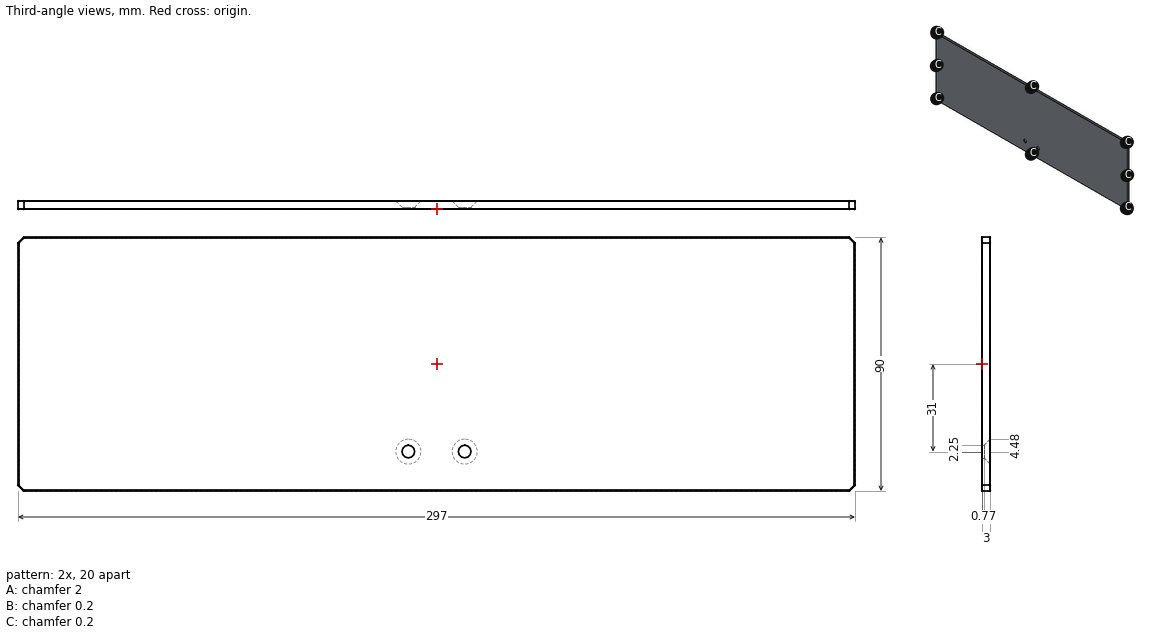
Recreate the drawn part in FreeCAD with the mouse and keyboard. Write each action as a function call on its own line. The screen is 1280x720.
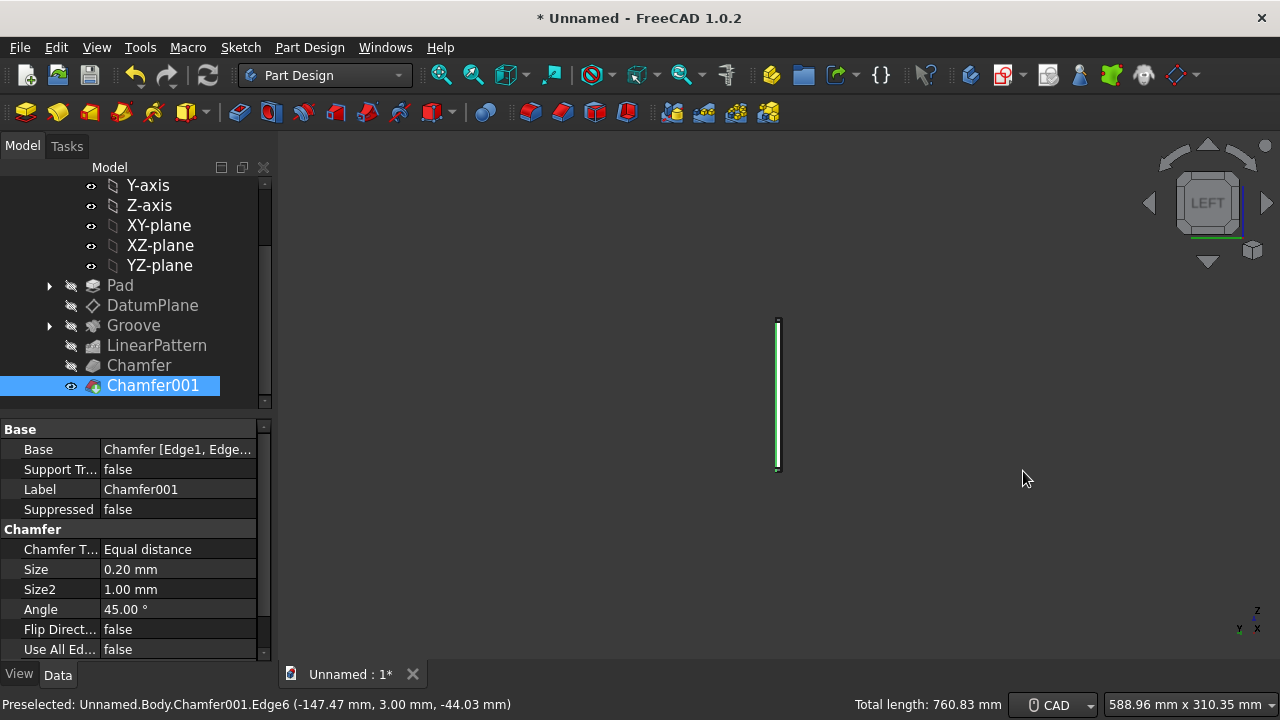
scroll(776, 319, up, 11)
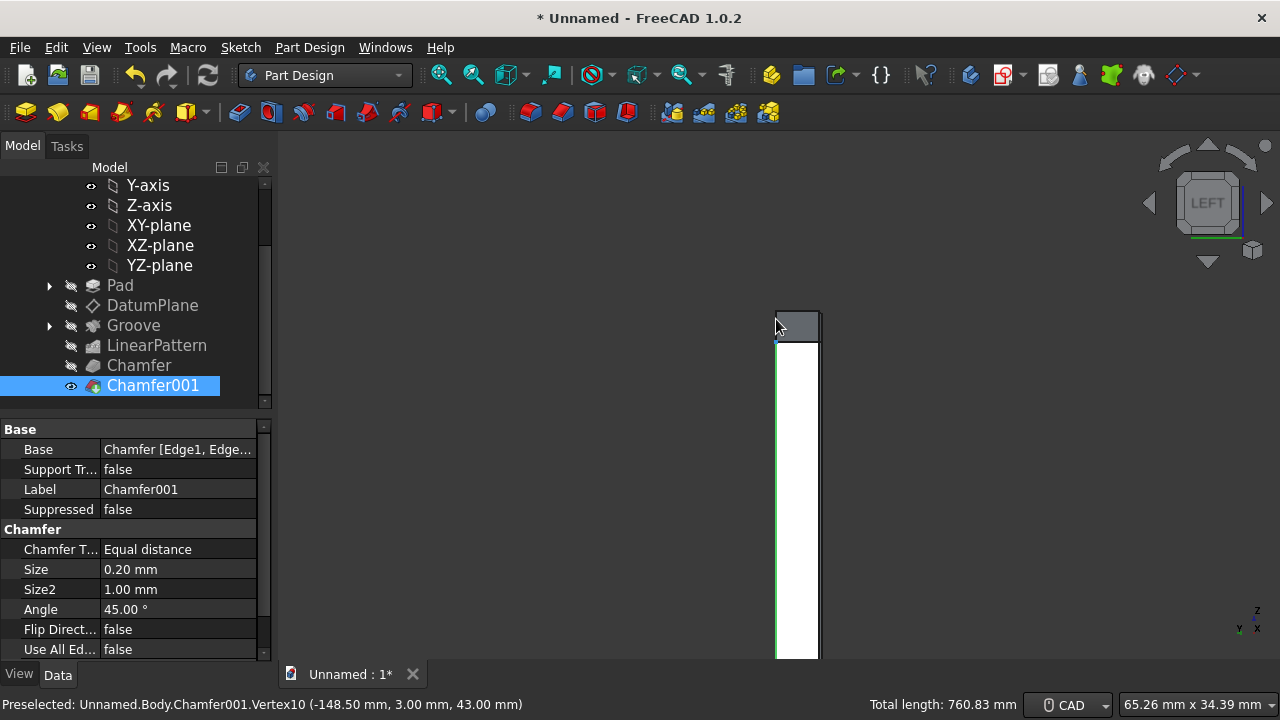
click(776, 325, ctrl)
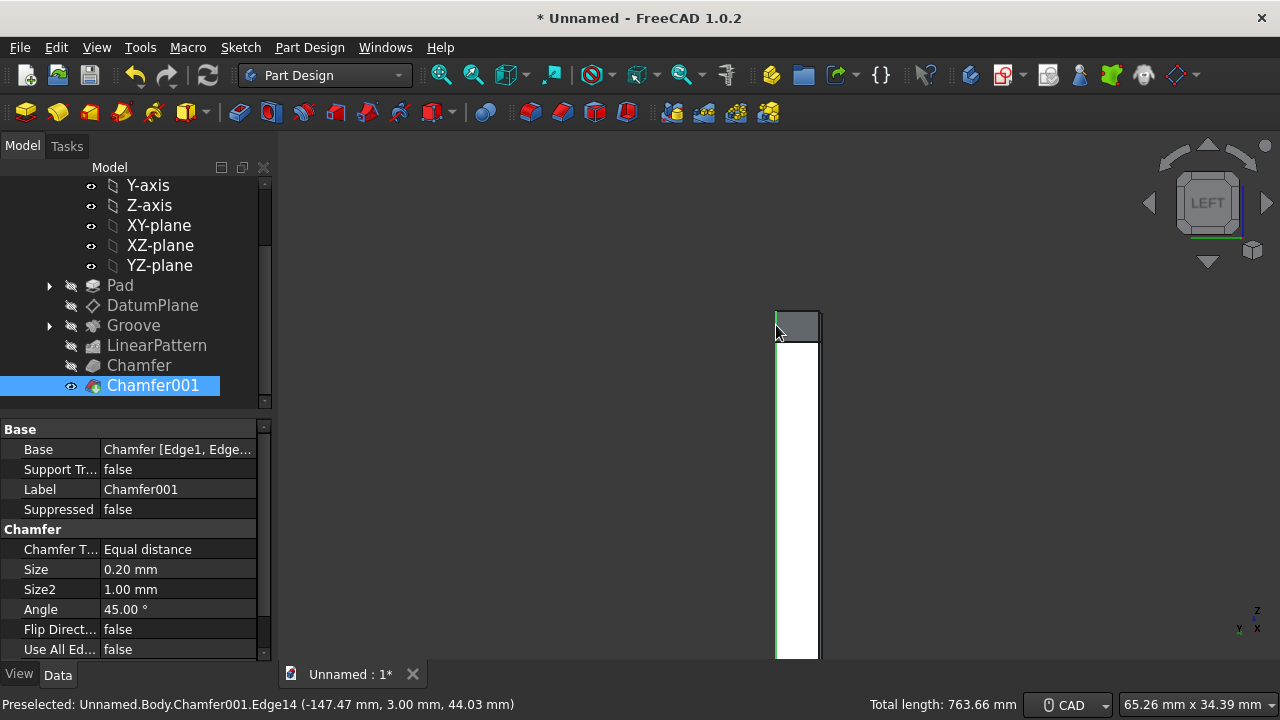
key(v)
key(f)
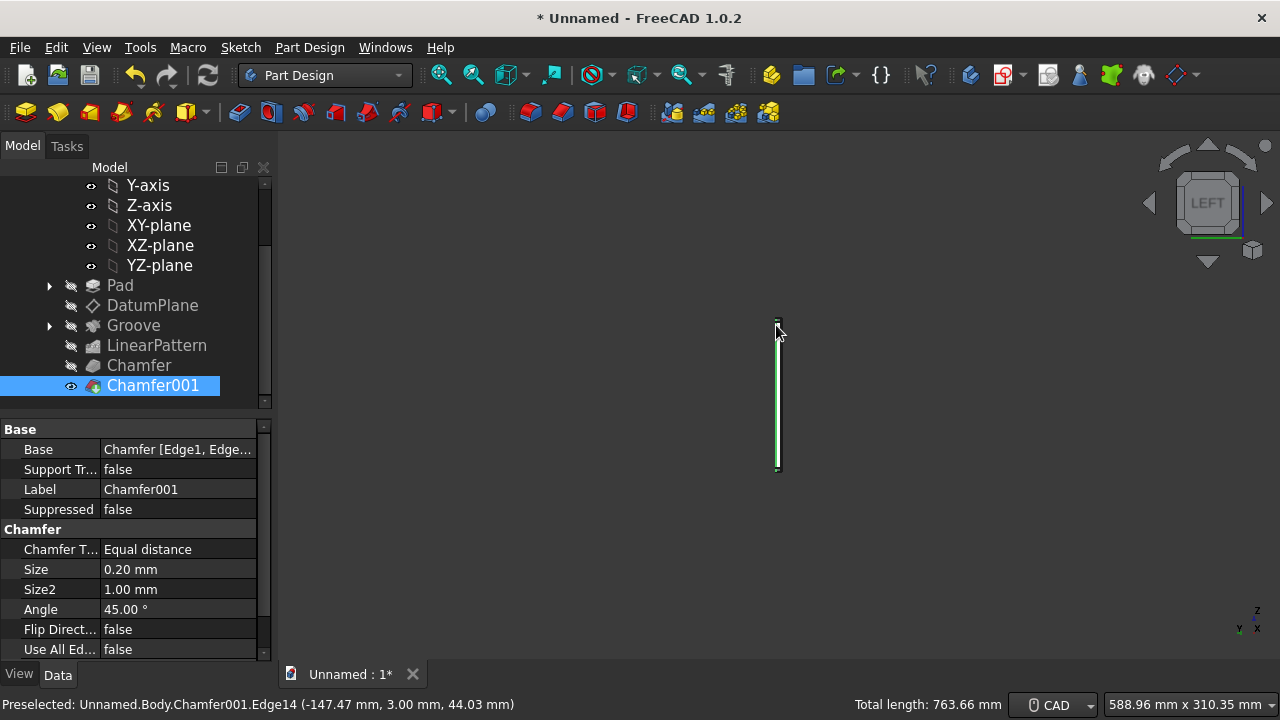
key(v)
key(3)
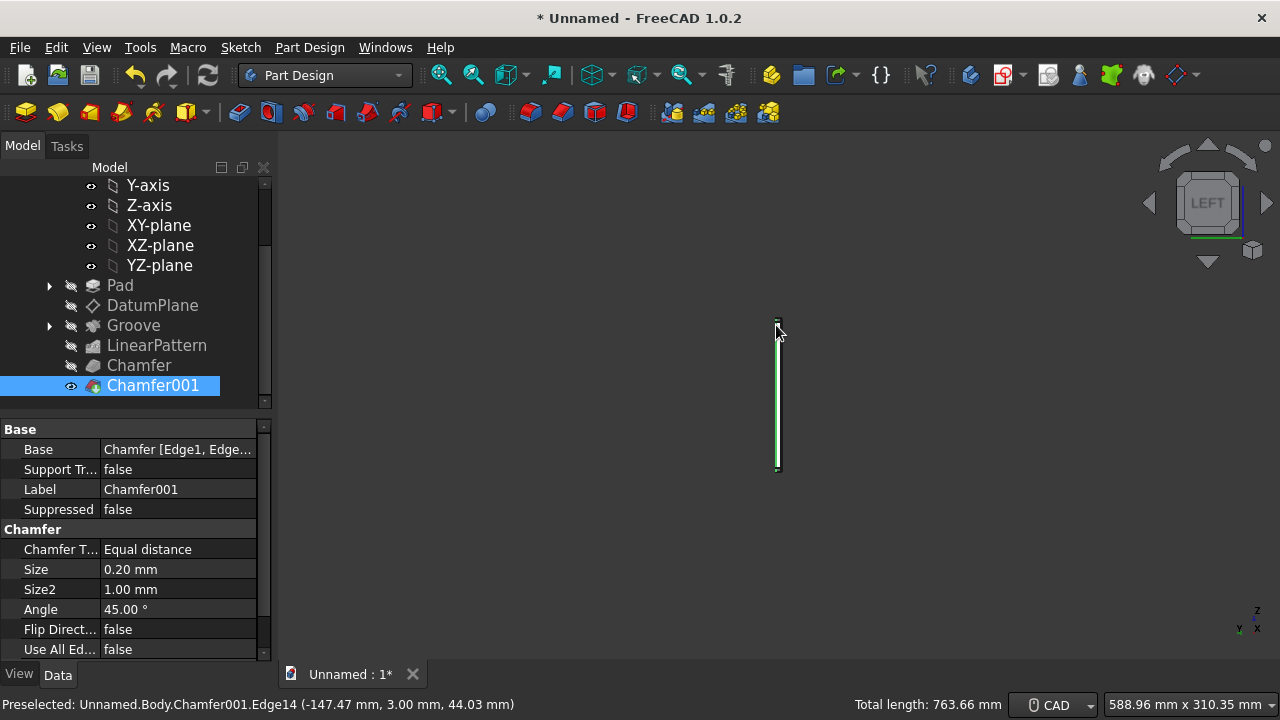
key(0)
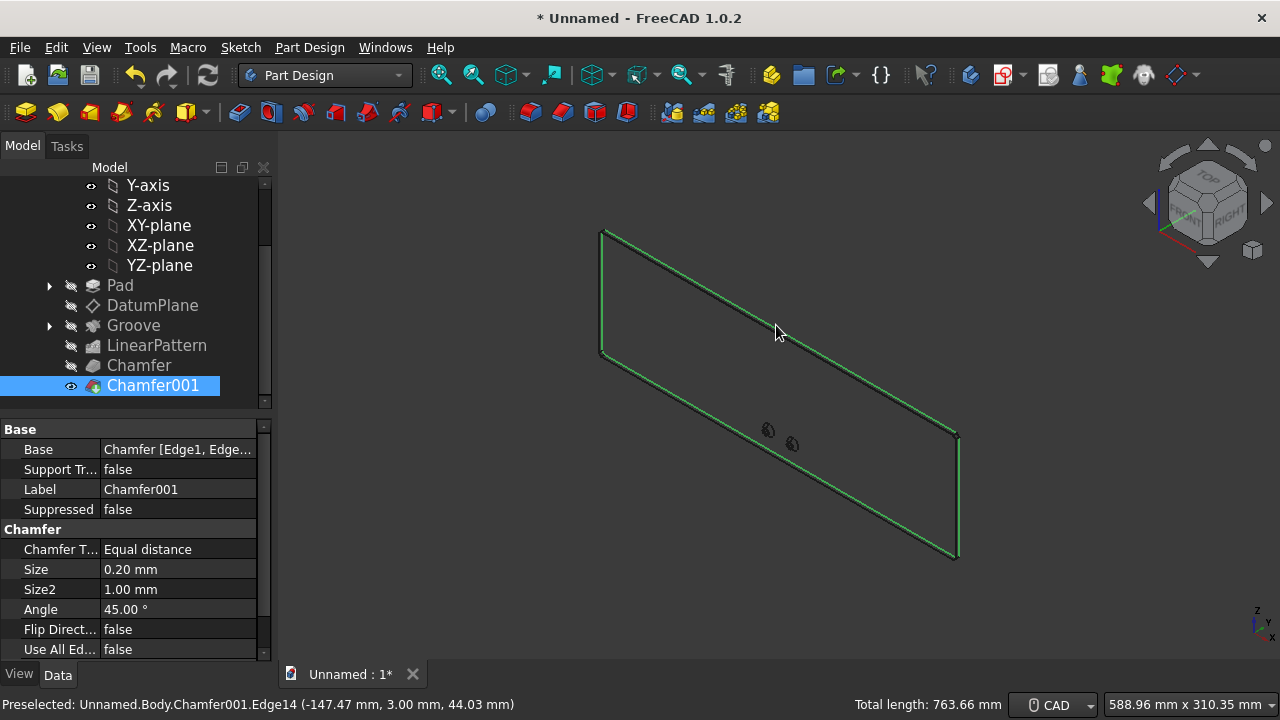
scroll(958, 434, up, 11)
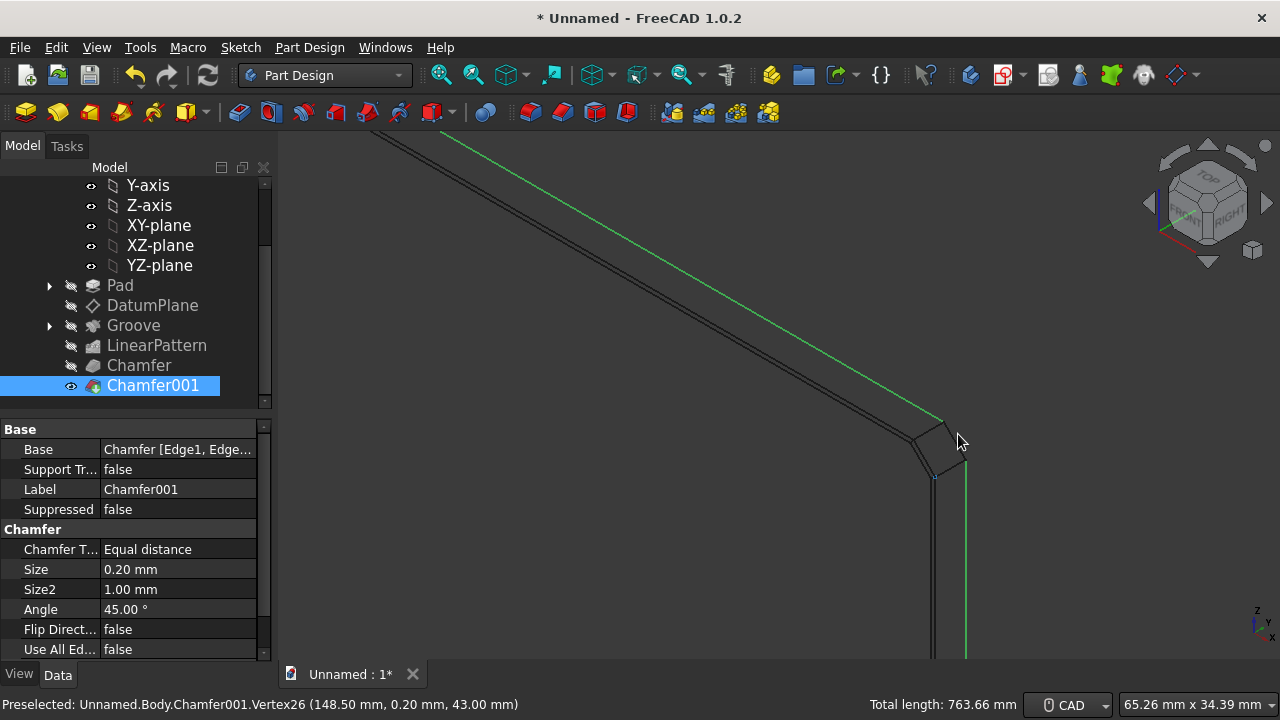
click(955, 440, ctrl)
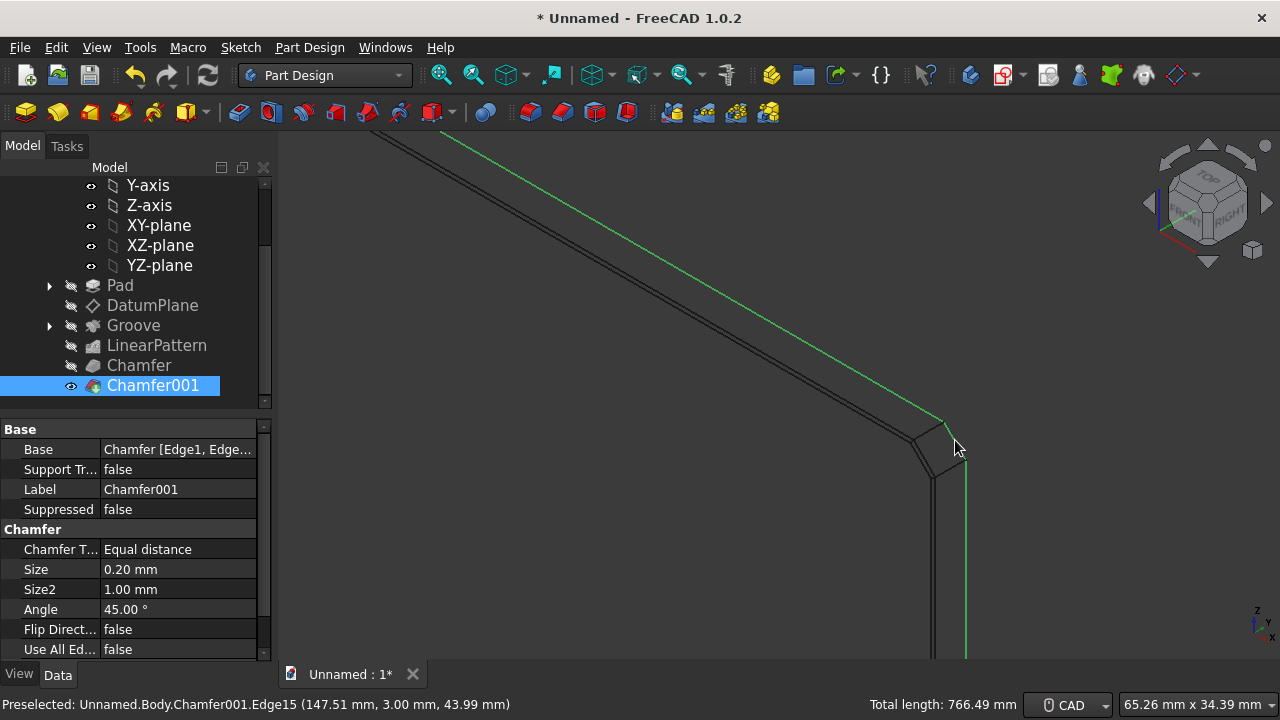
key(v)
key(f)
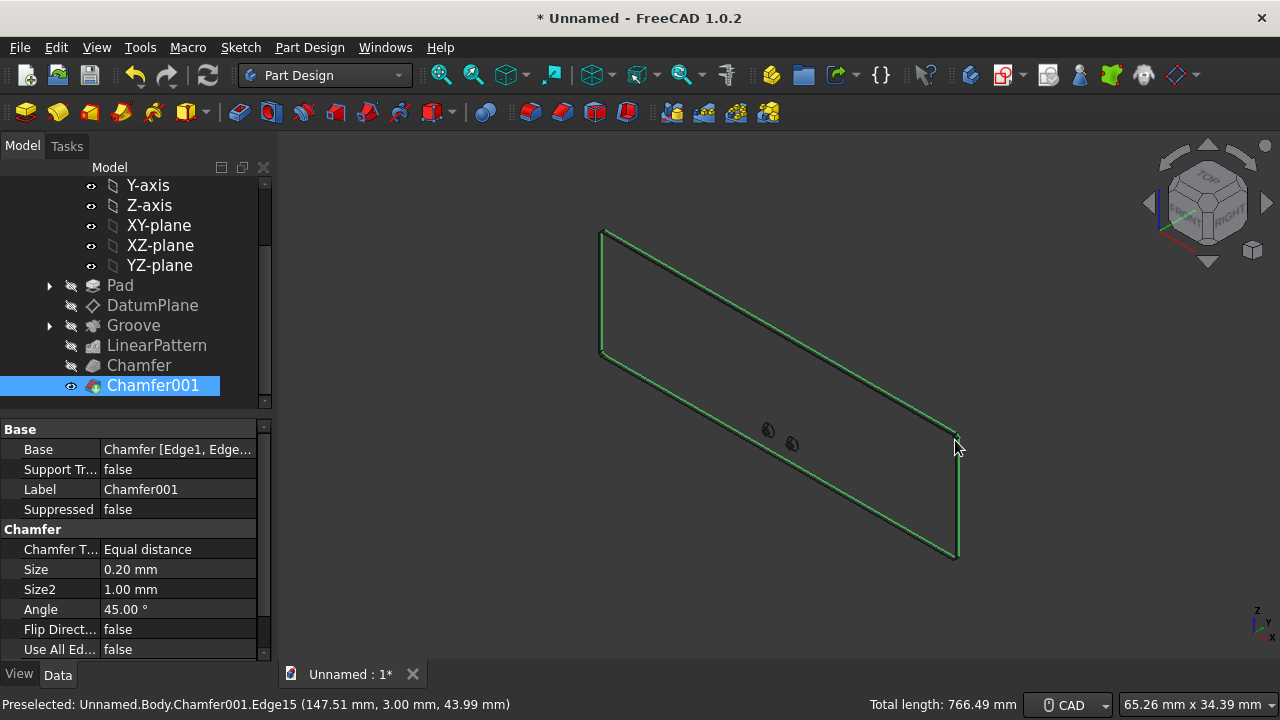
key(2)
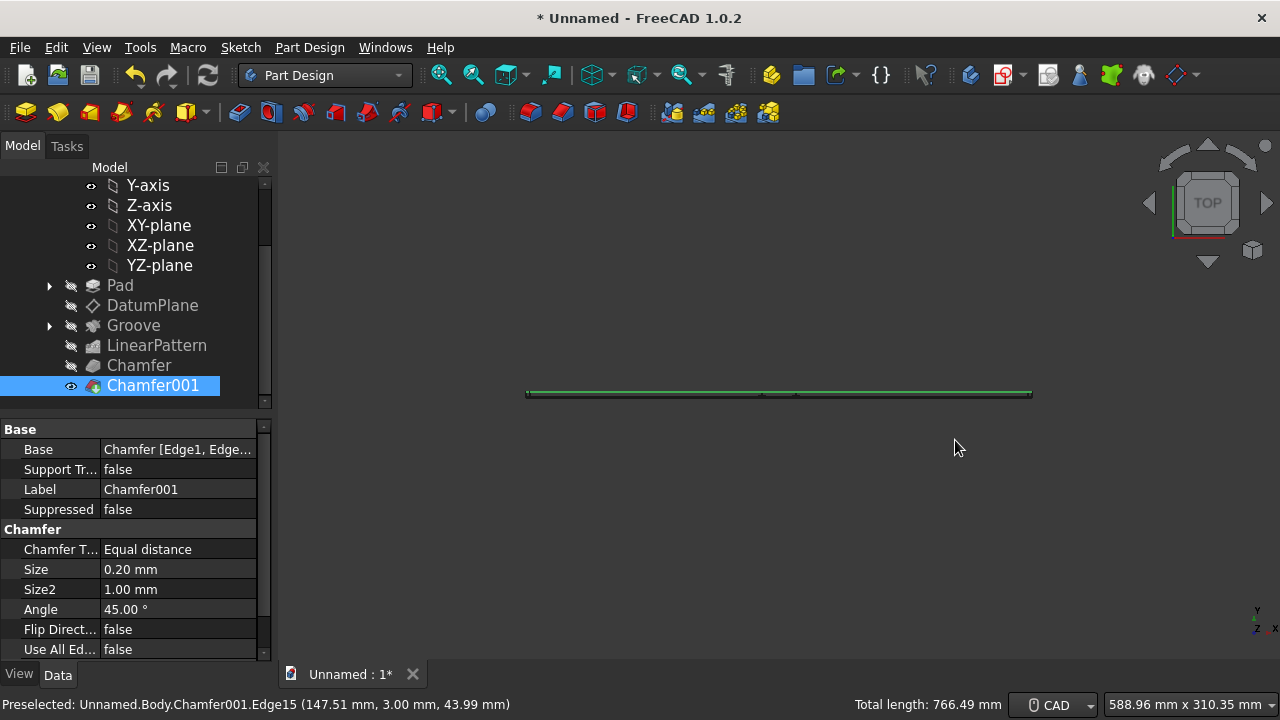
scroll(1030, 391, up, 11)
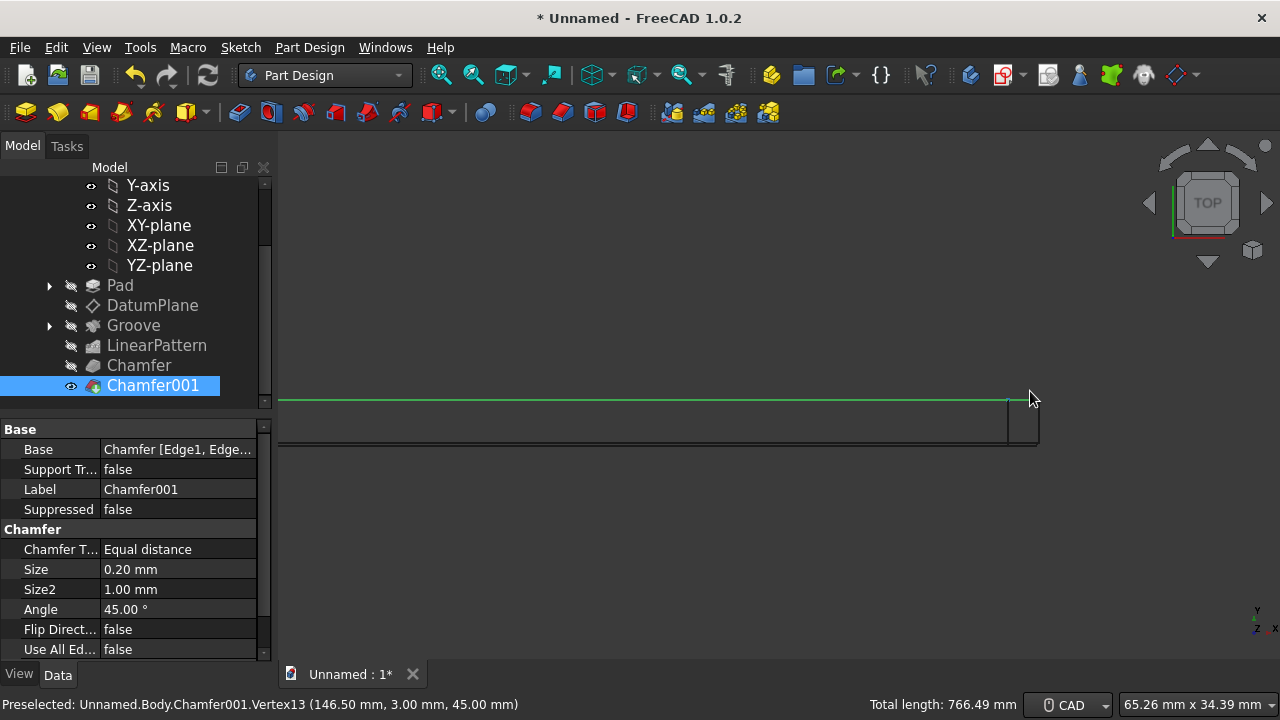
click(442, 76)